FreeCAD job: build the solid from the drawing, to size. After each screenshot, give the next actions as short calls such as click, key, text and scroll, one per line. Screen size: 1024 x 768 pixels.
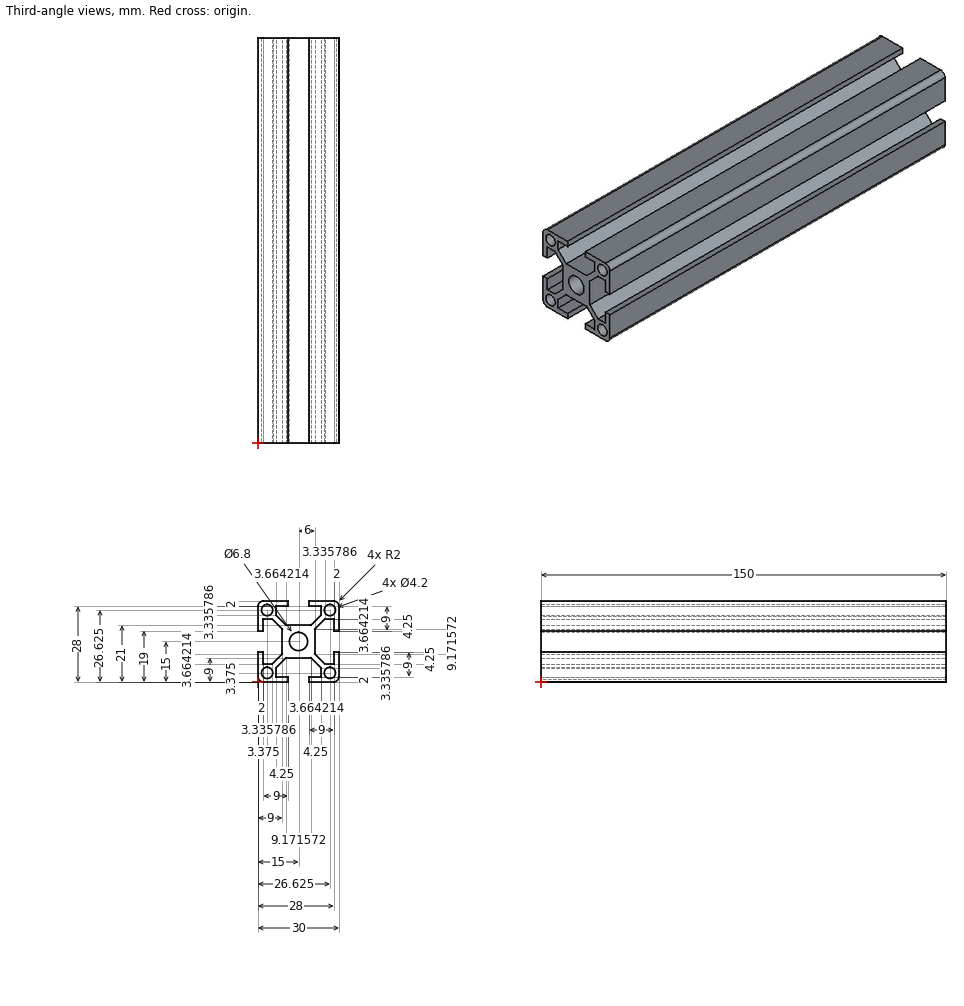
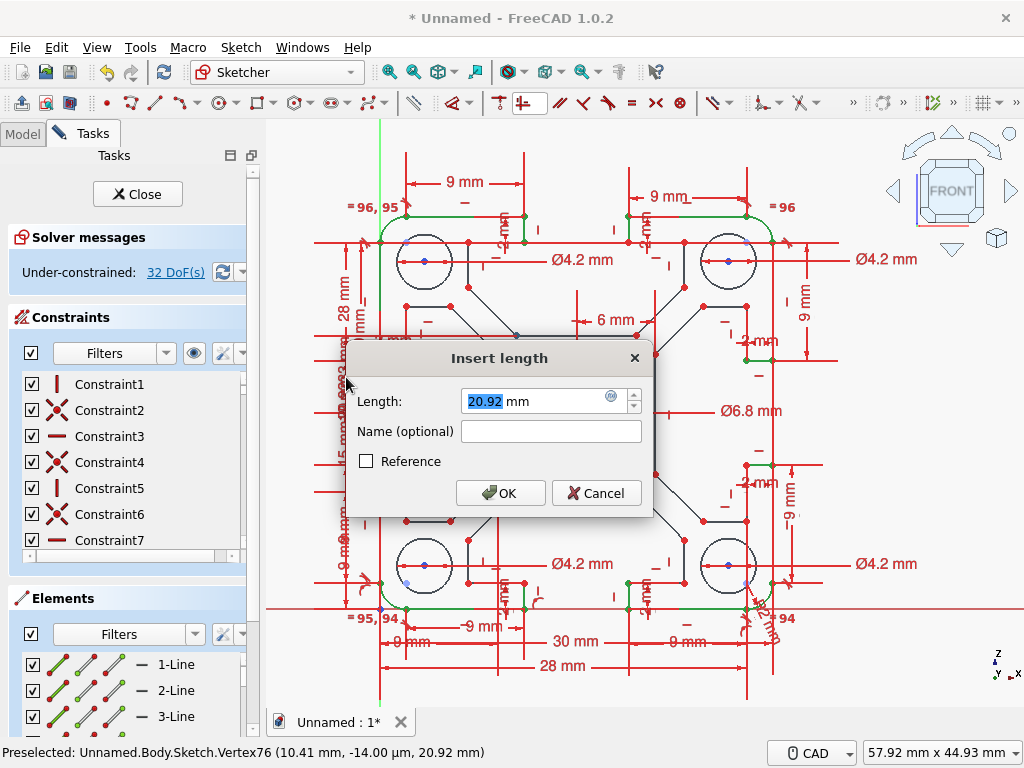
text(21)
key(Return)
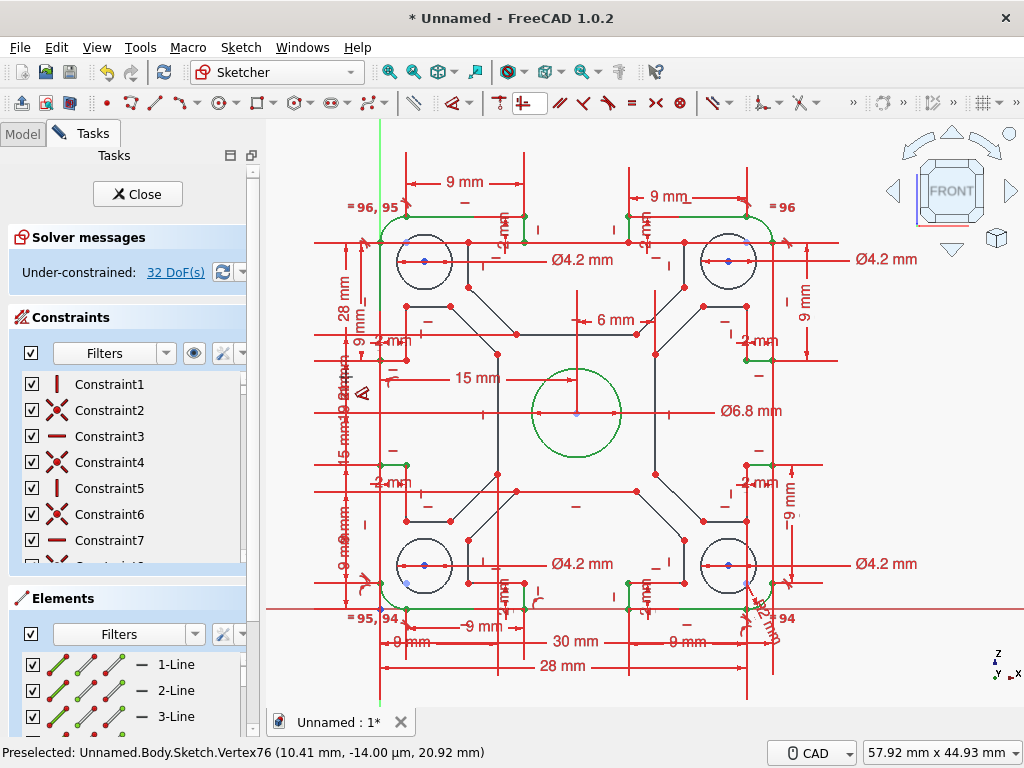
click(747, 344)
click(713, 321)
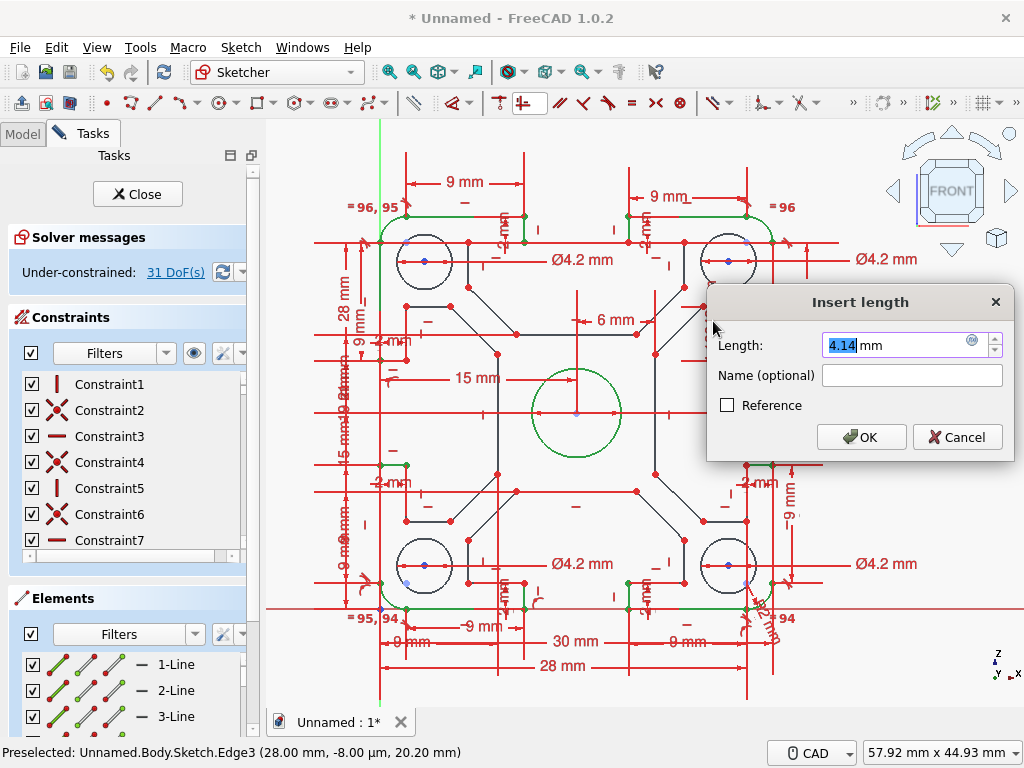
text(4.25)
key(Return)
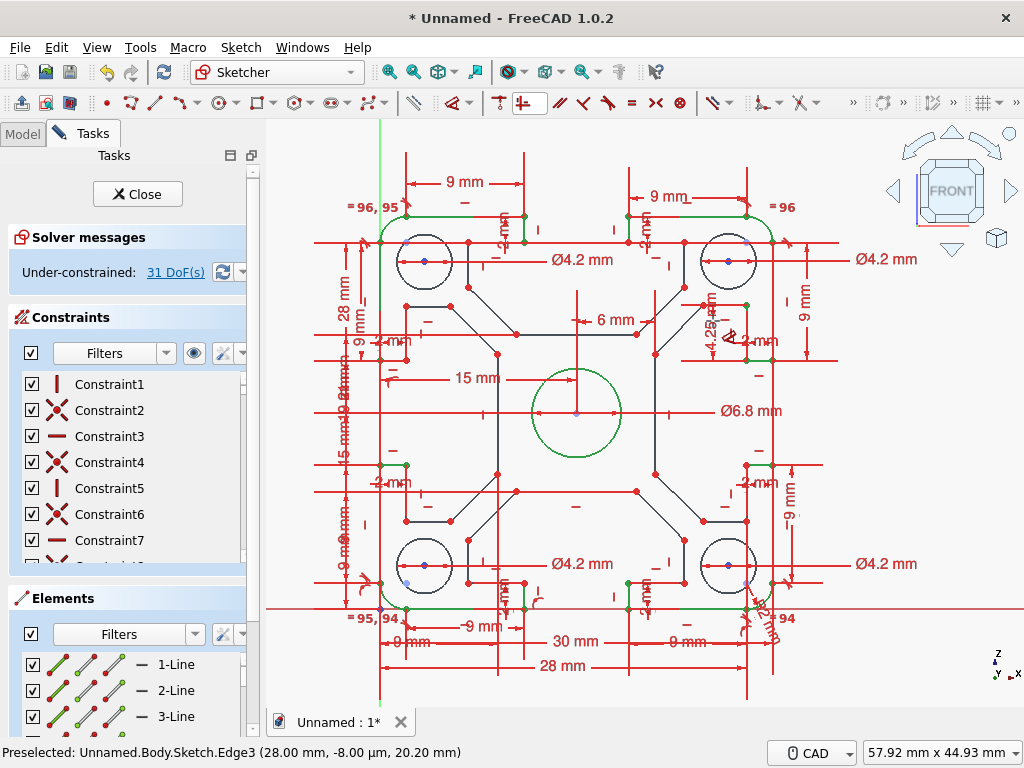
click(747, 505)
click(713, 506)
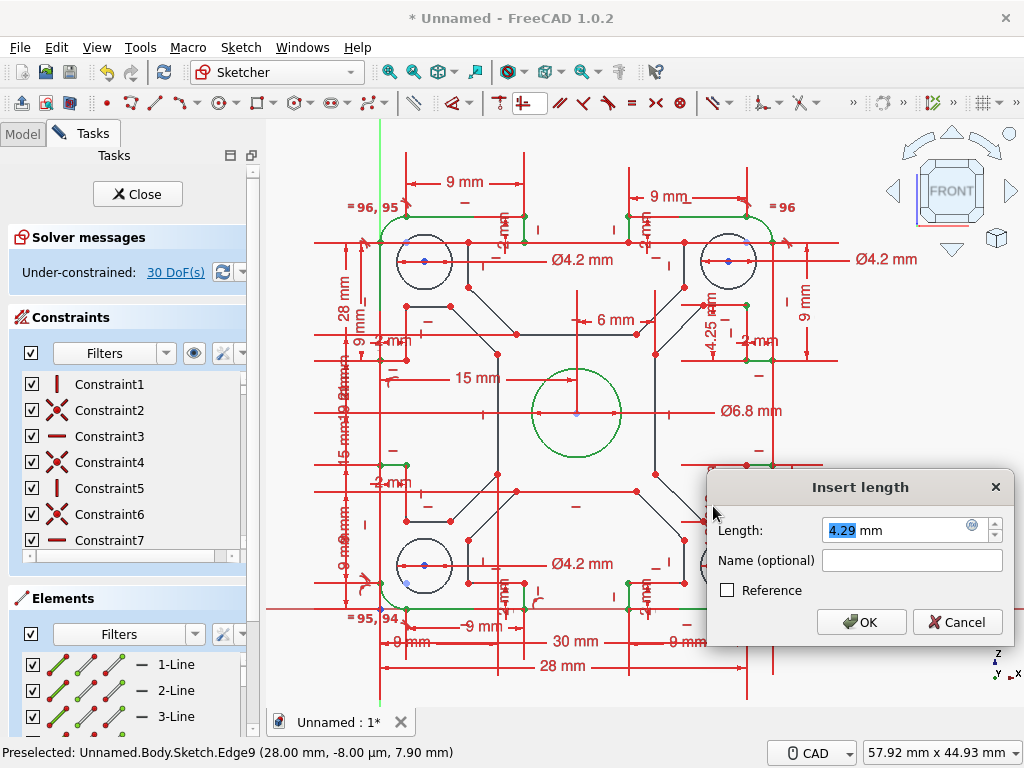
text(4.25)
key(Return)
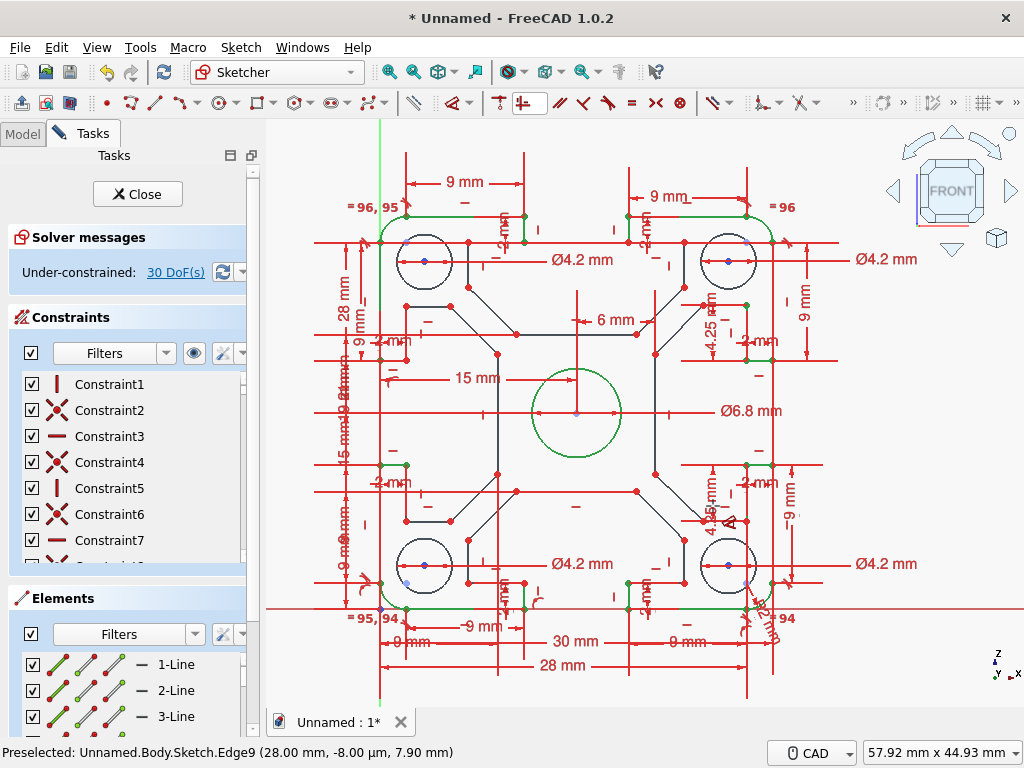
click(646, 583)
click(657, 549)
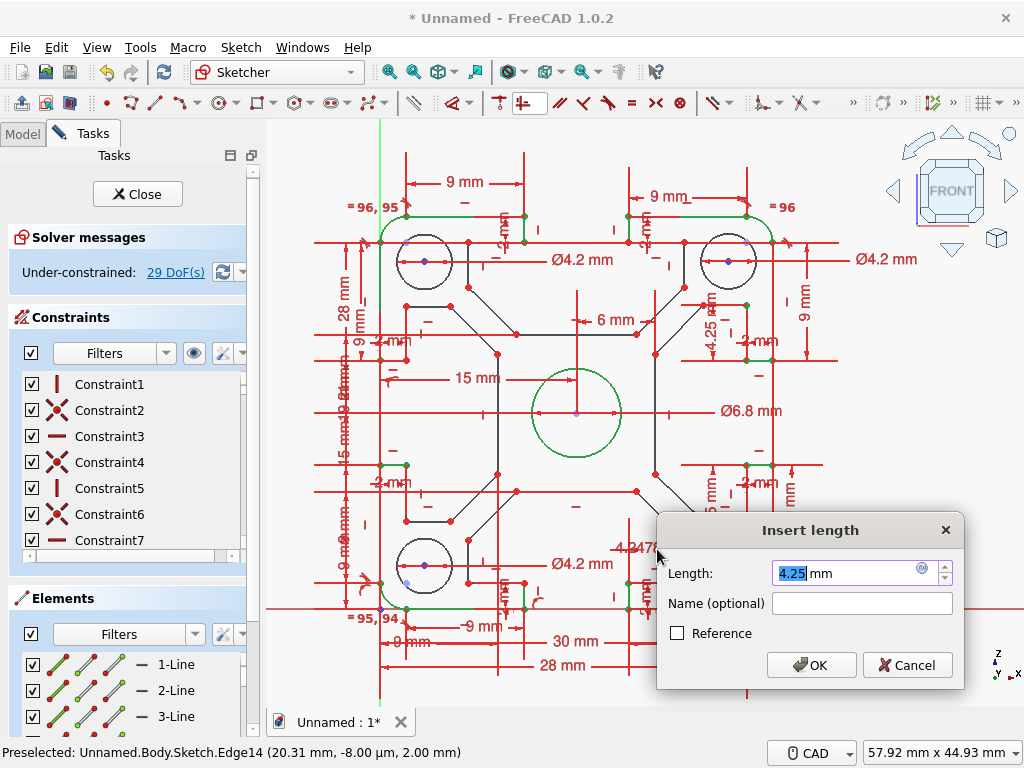
text(4.25)
key(Return)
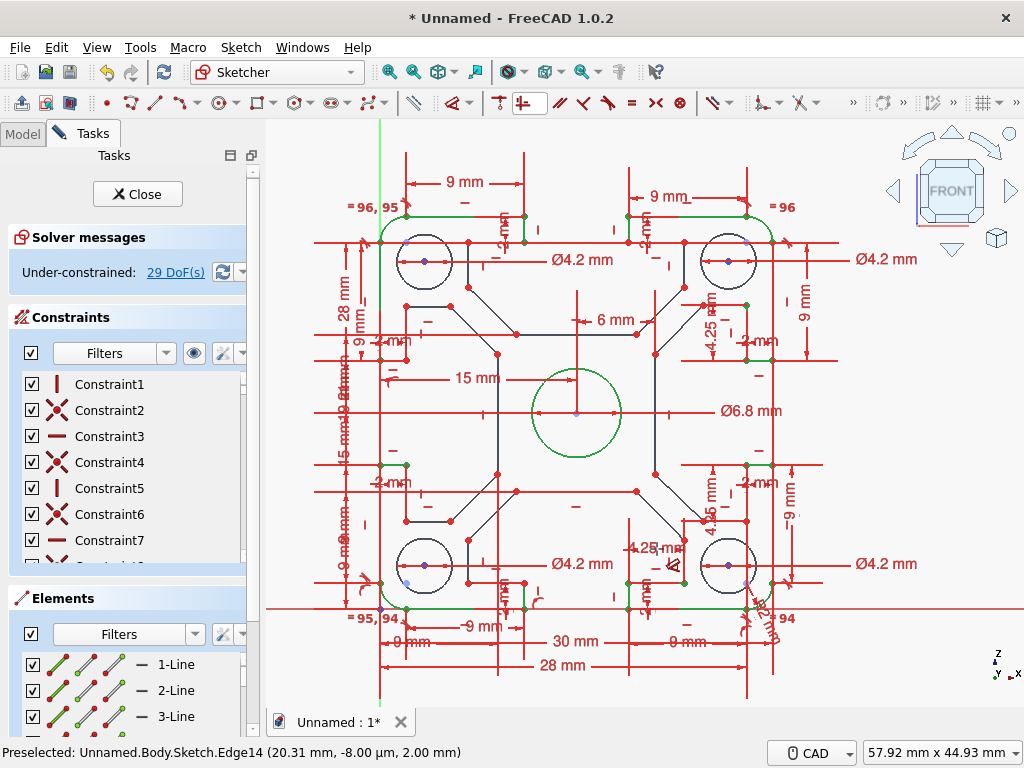
click(485, 583)
click(496, 549)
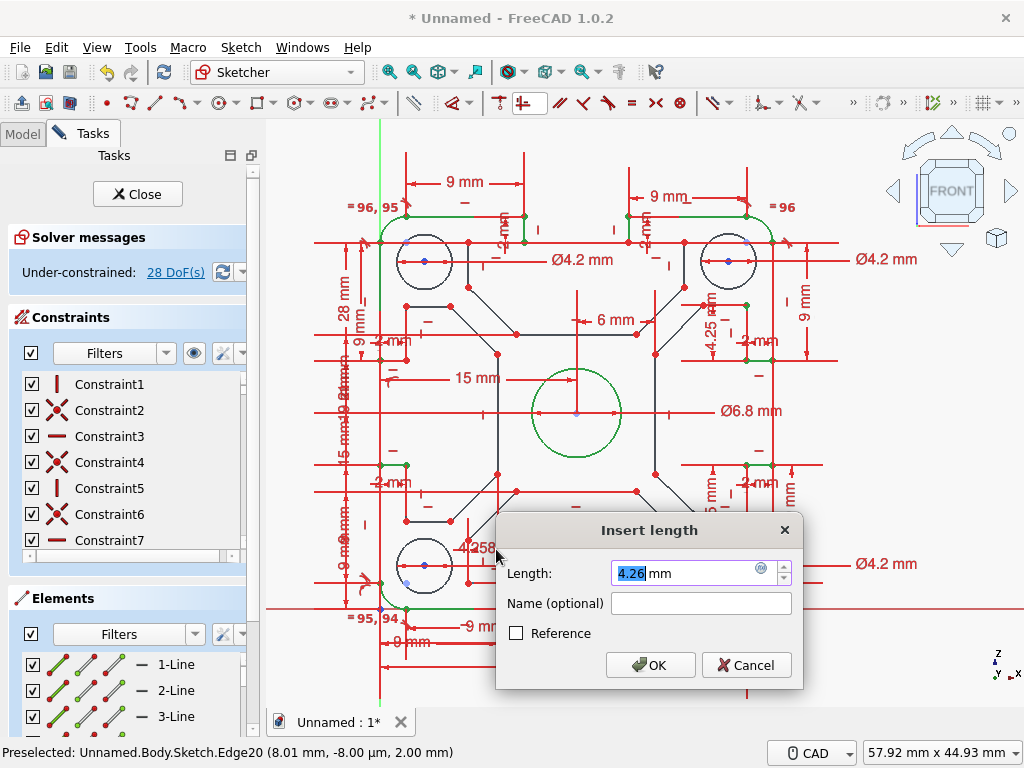
text(4.25)
key(Return)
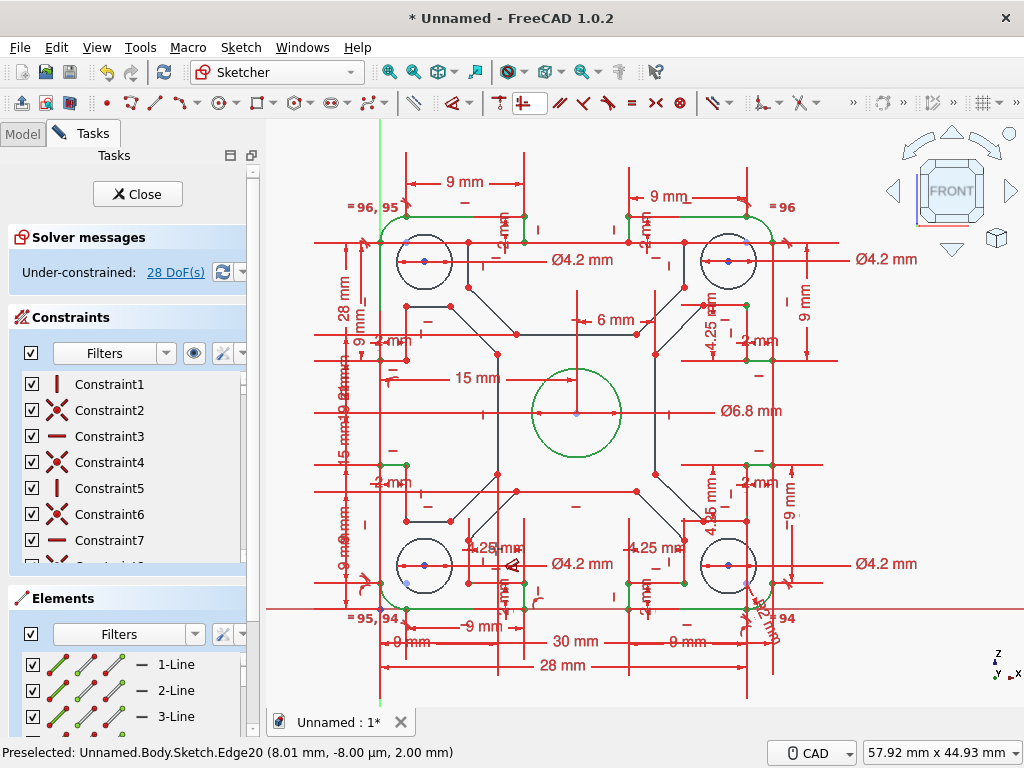
click(406, 482)
click(440, 506)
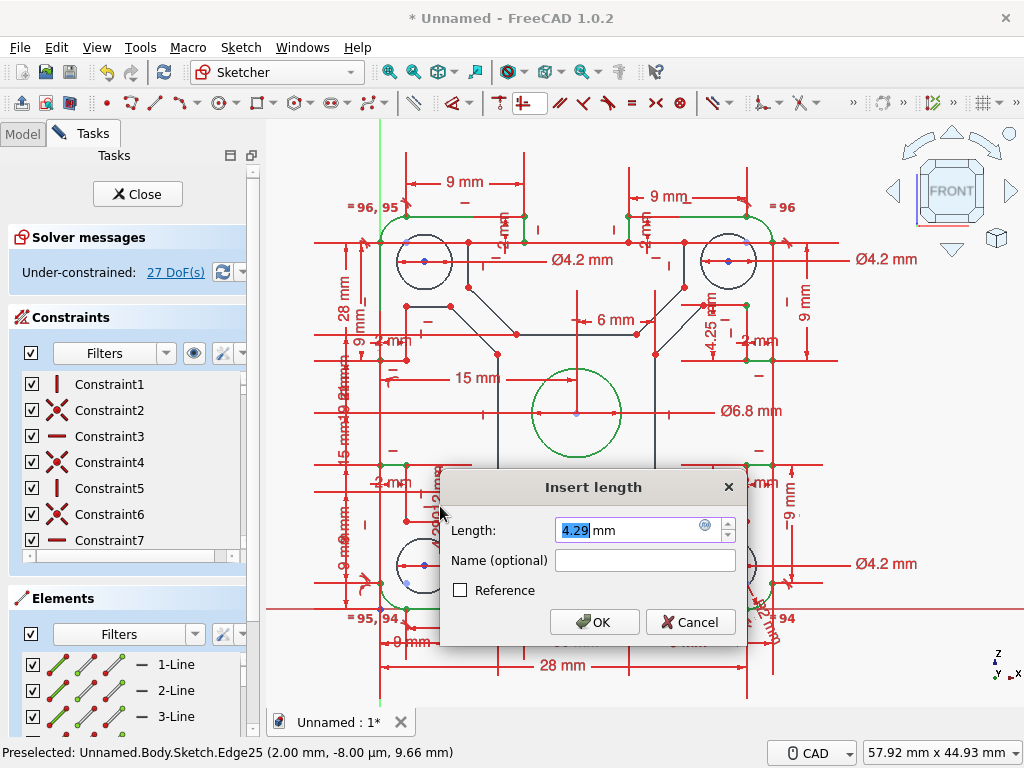
text(4.25)
key(Return)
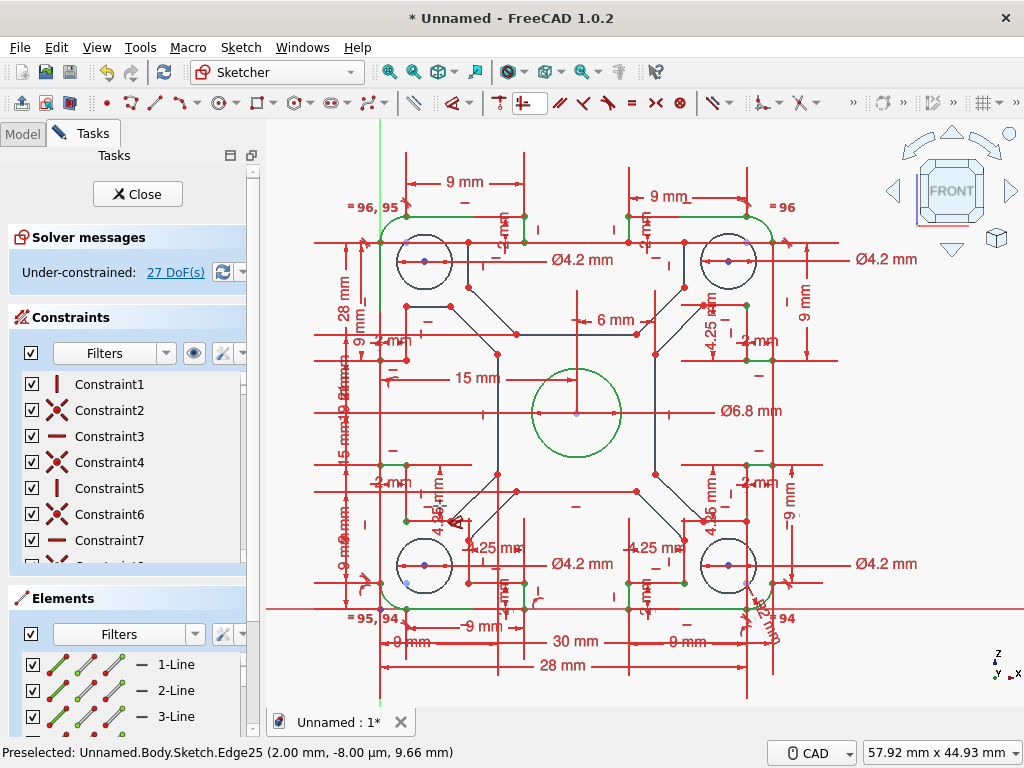
click(406, 323)
click(440, 321)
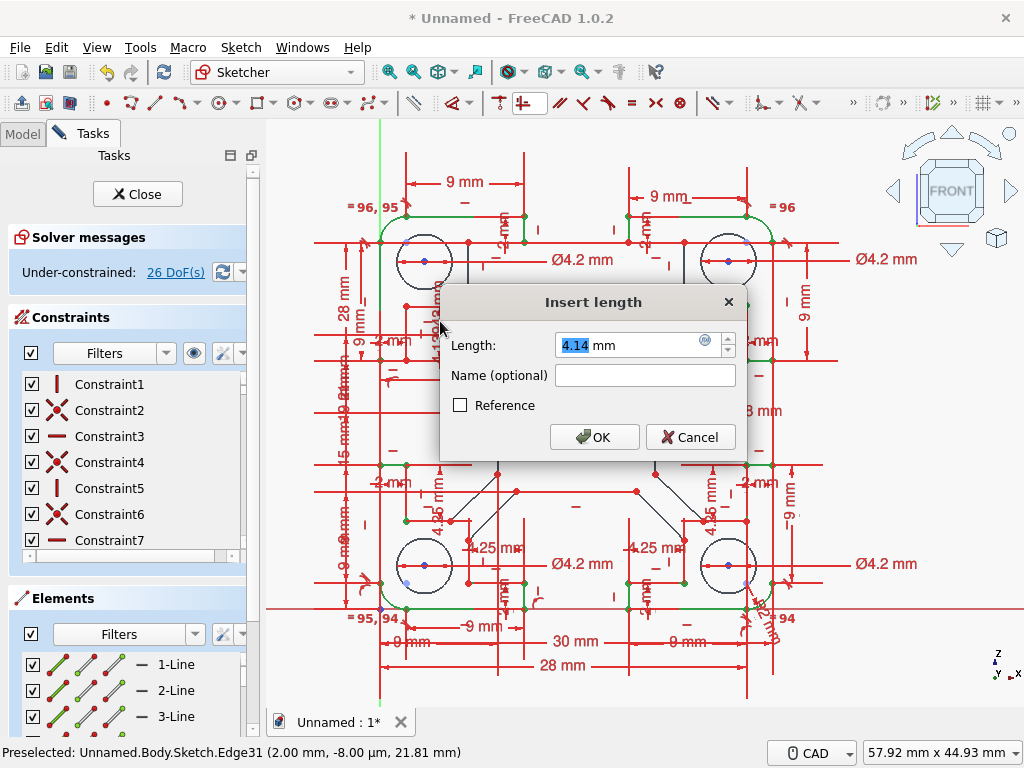
text(4.25)
key(Return)